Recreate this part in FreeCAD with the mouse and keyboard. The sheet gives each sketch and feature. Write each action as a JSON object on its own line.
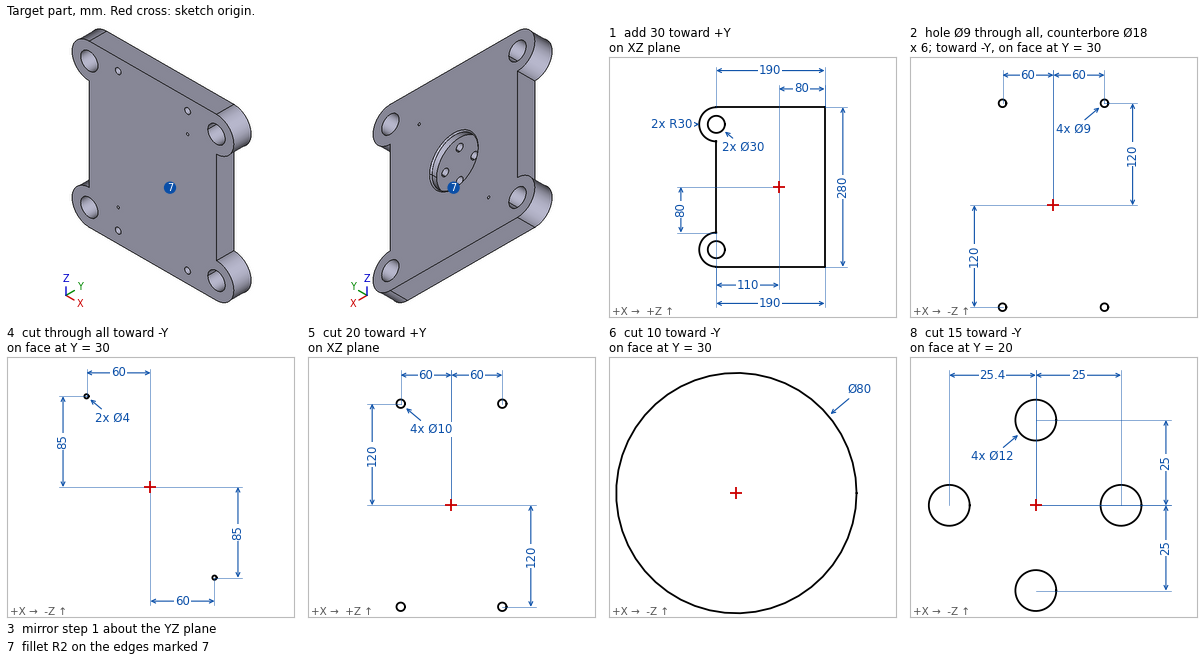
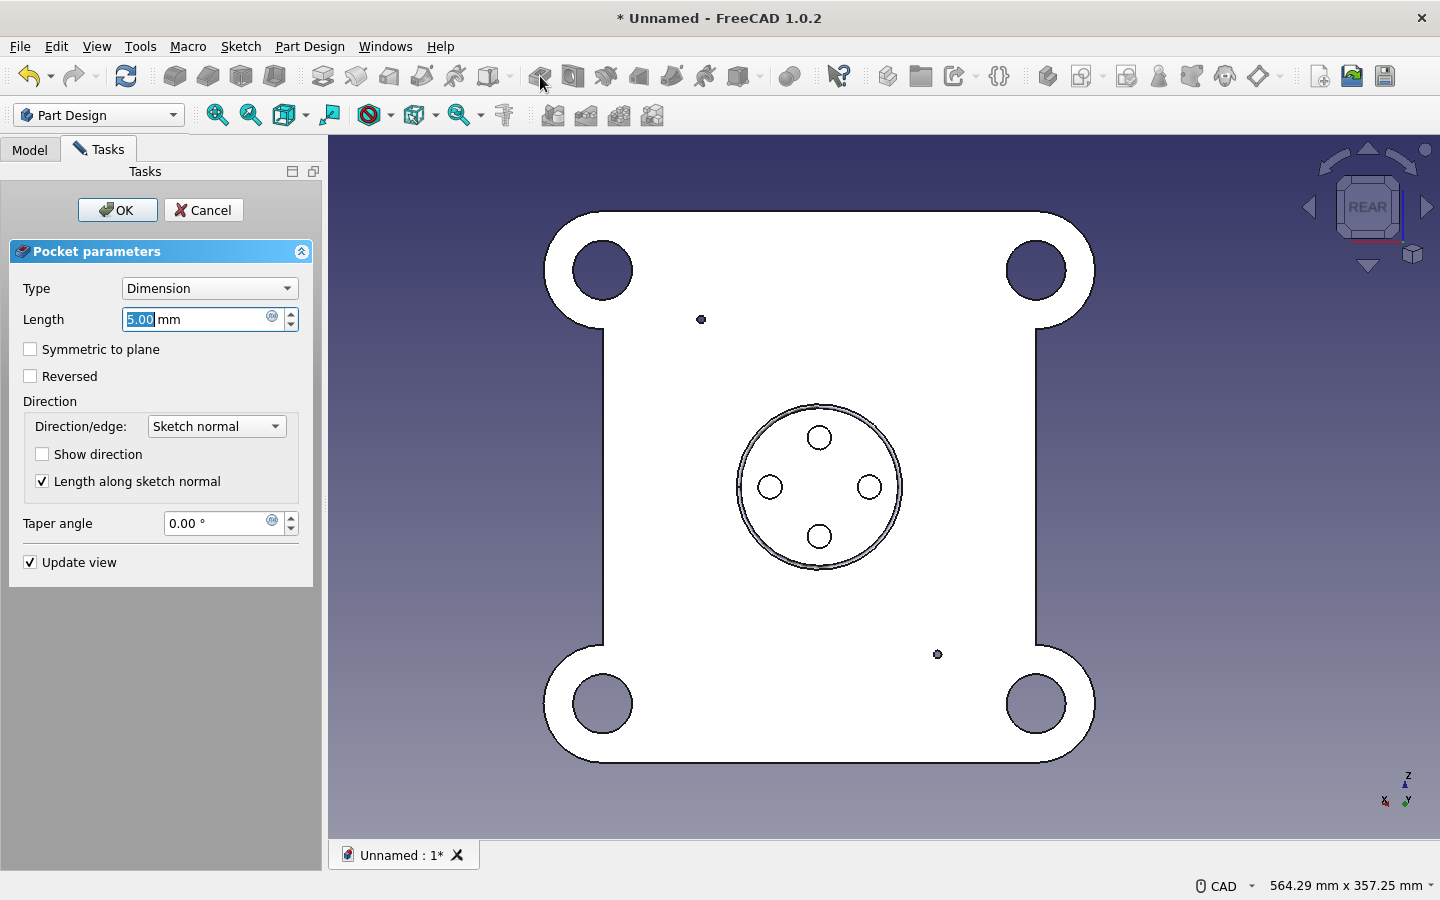
{"action": "type", "text": "15"}
{"action": "key", "text": "Tab"}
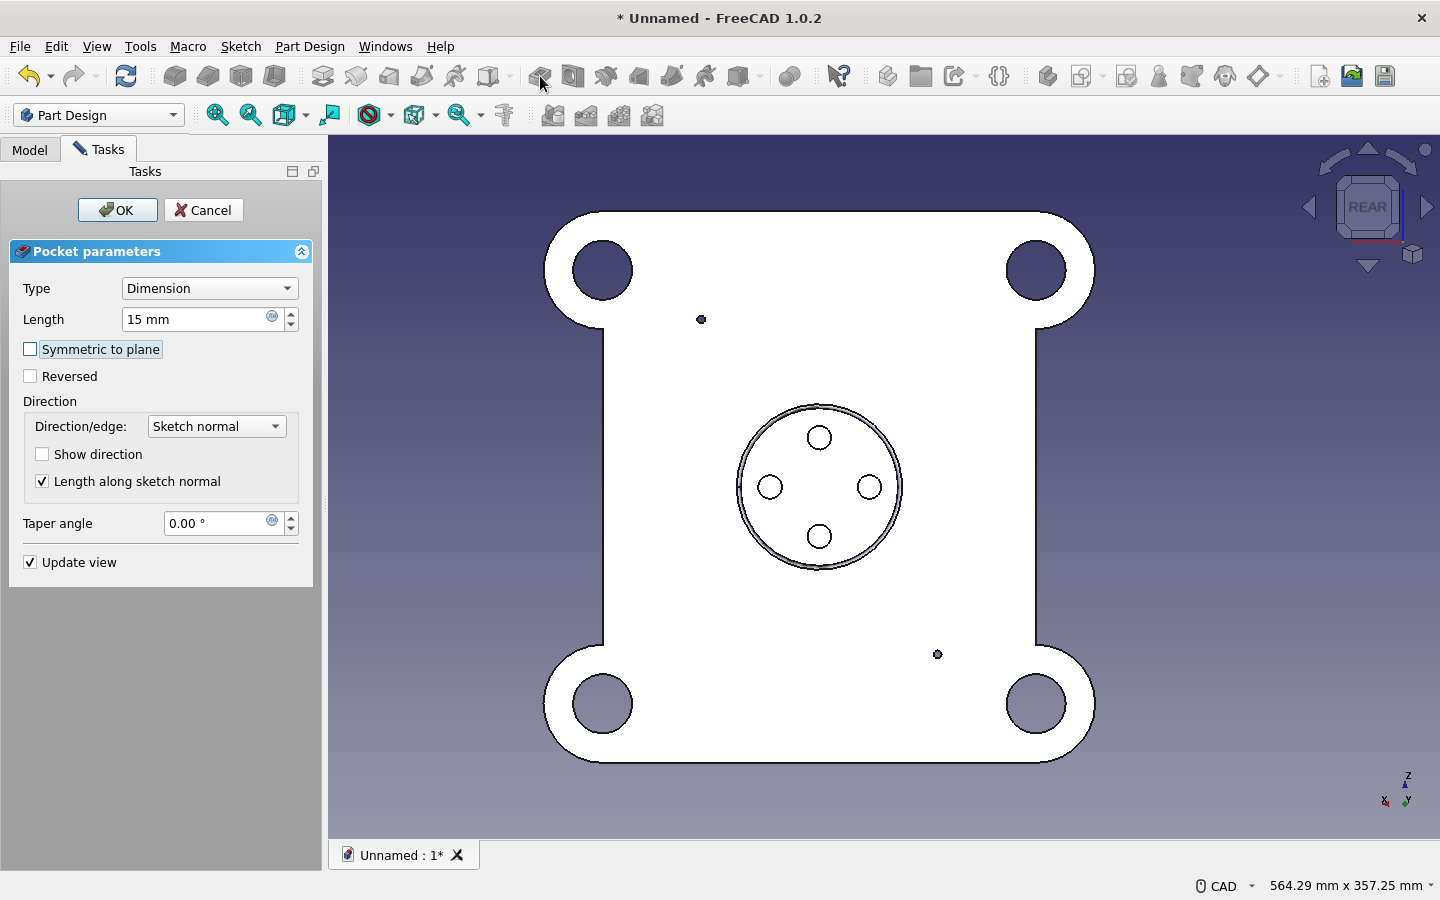
{"action": "left_click", "coordinate": [118, 210]}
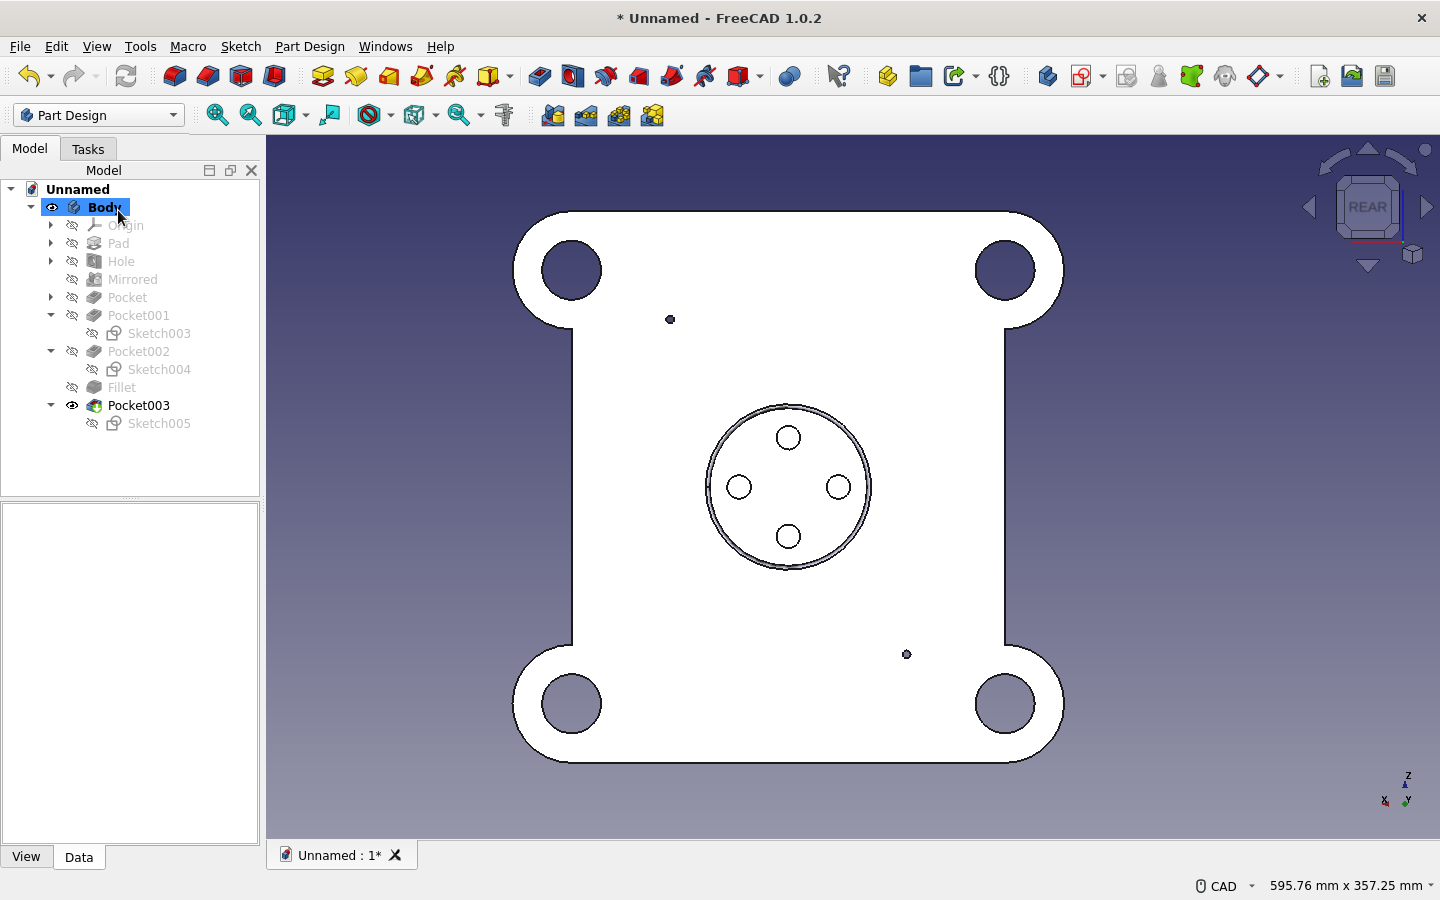
{"action": "key", "text": "0"}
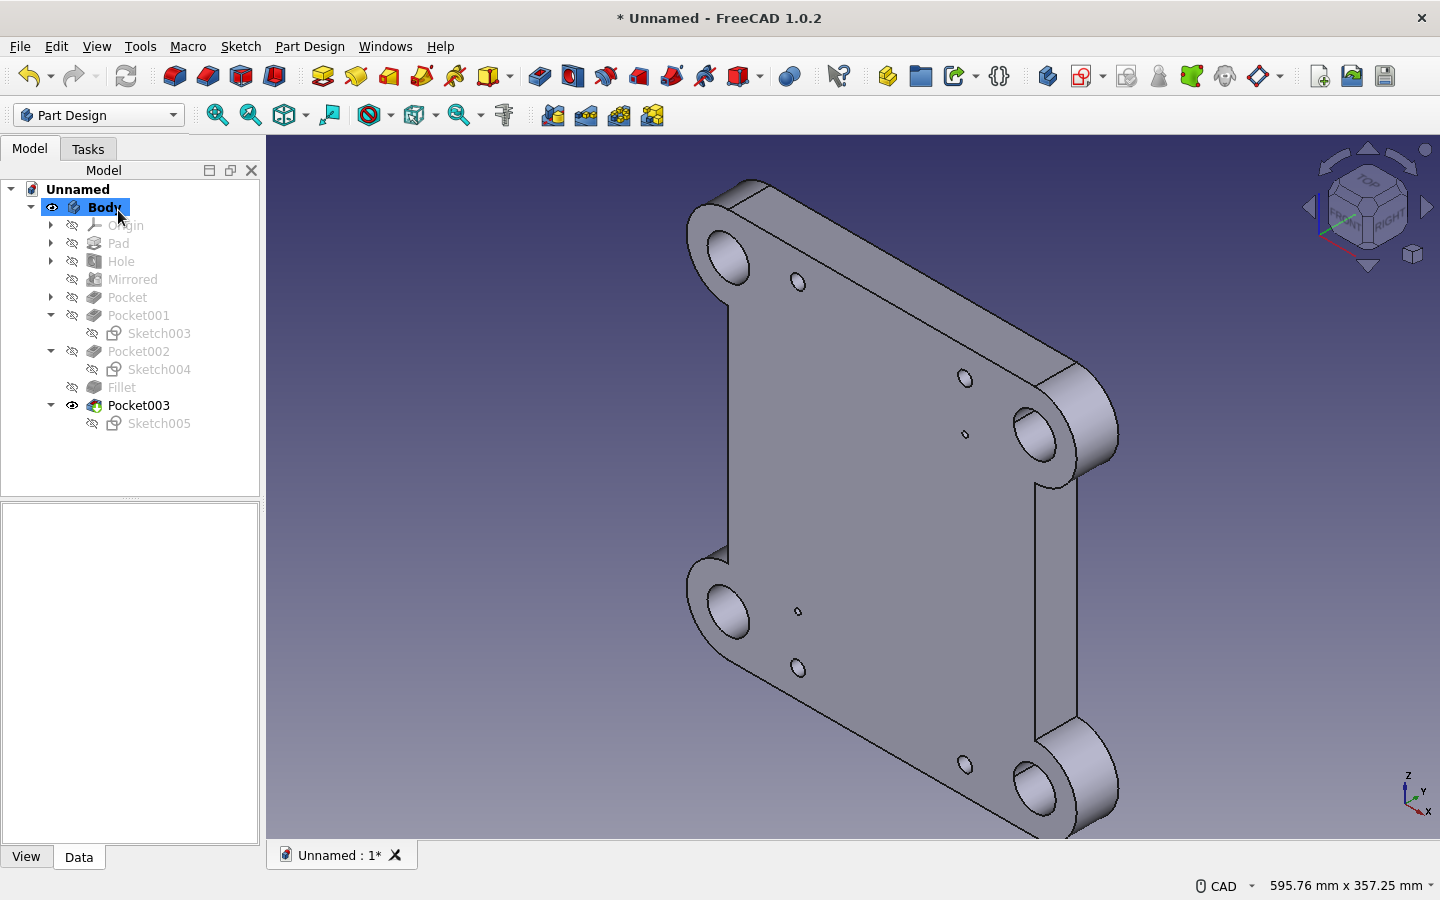
{"action": "left_click", "coordinate": [218, 116]}